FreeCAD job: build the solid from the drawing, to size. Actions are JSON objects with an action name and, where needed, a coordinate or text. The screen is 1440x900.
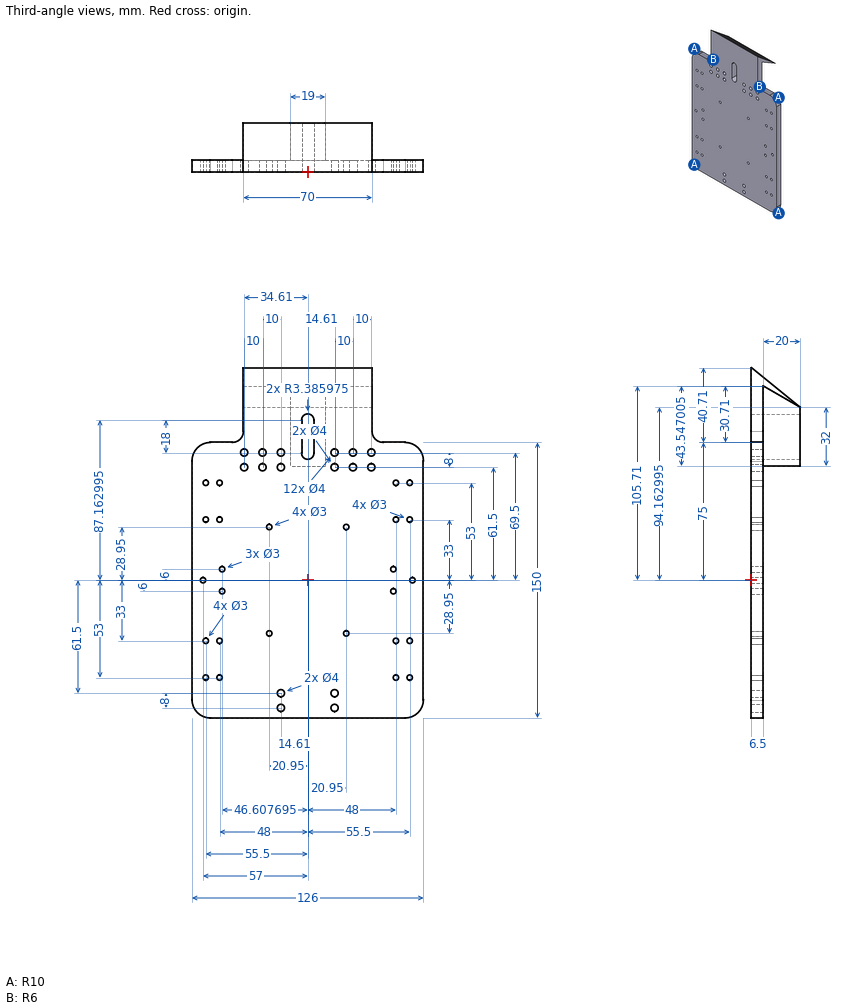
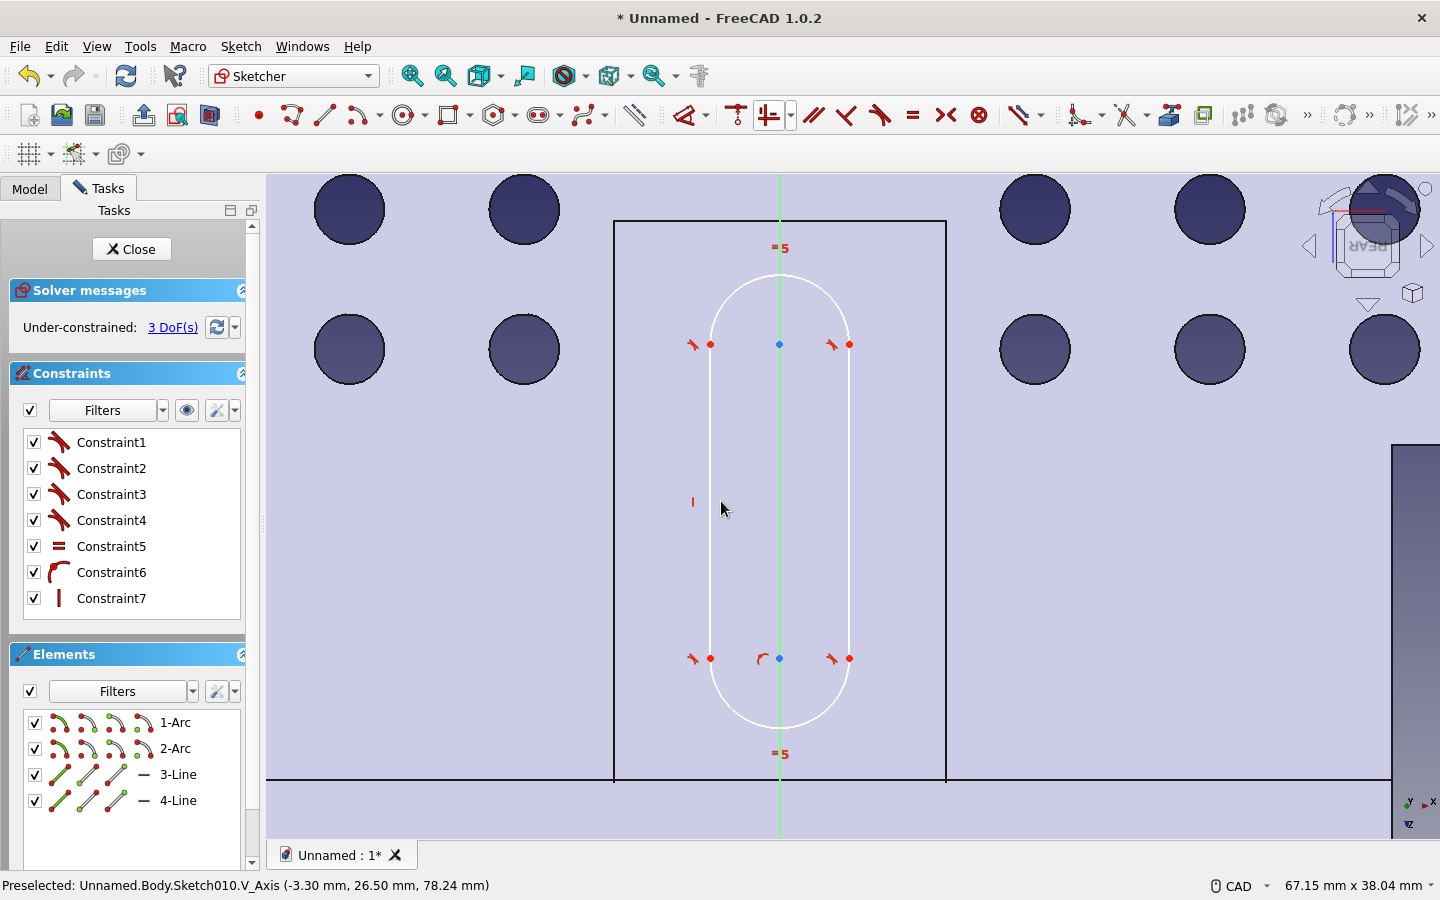
{"action": "left_click", "coordinate": [684, 116]}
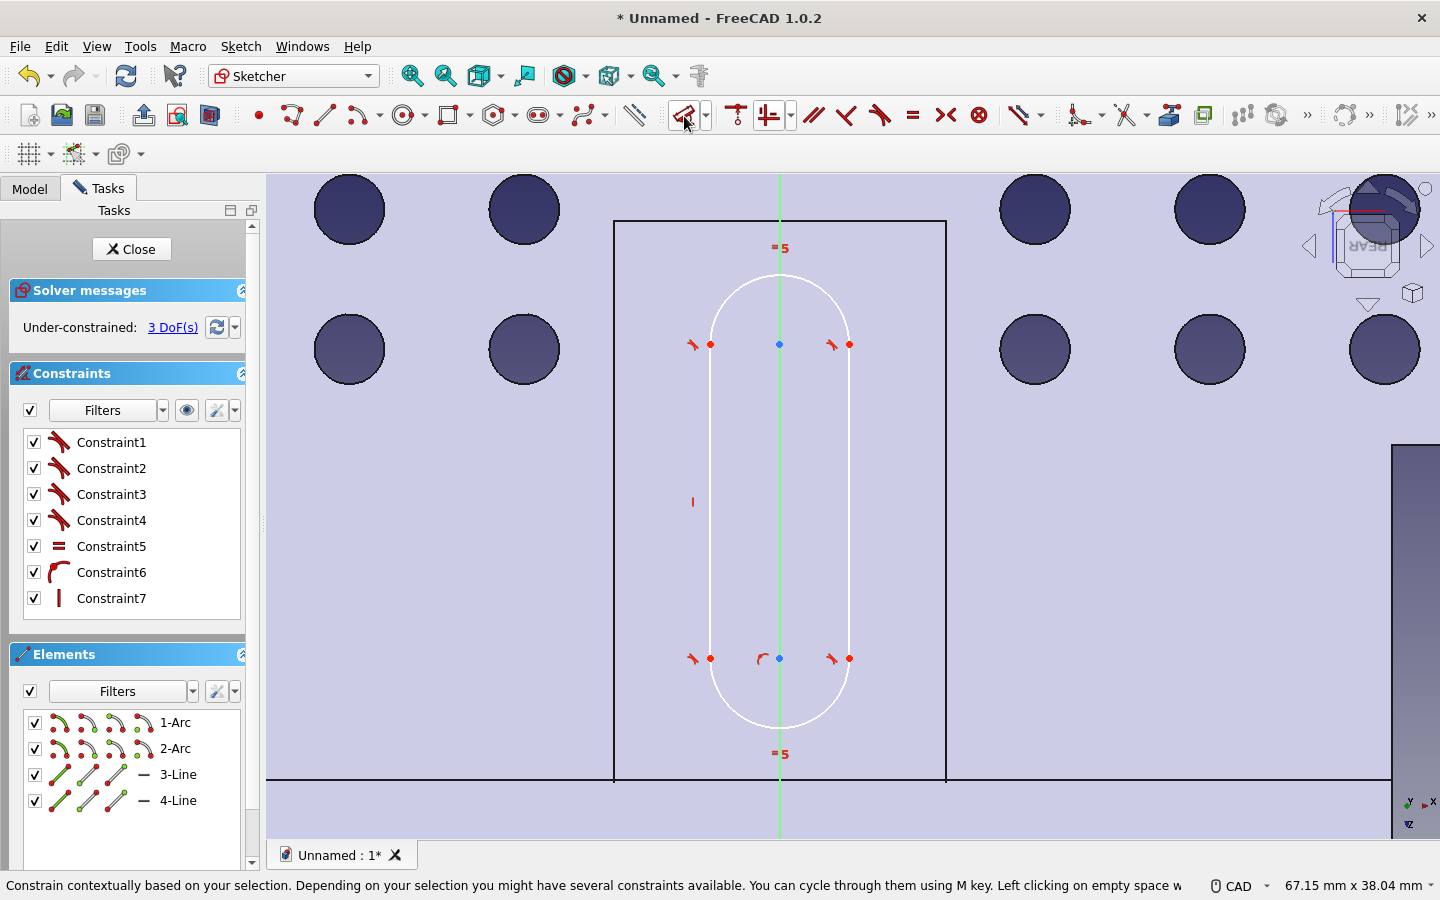
{"action": "left_click", "coordinate": [739, 715]}
{"action": "left_click", "coordinate": [720, 741]}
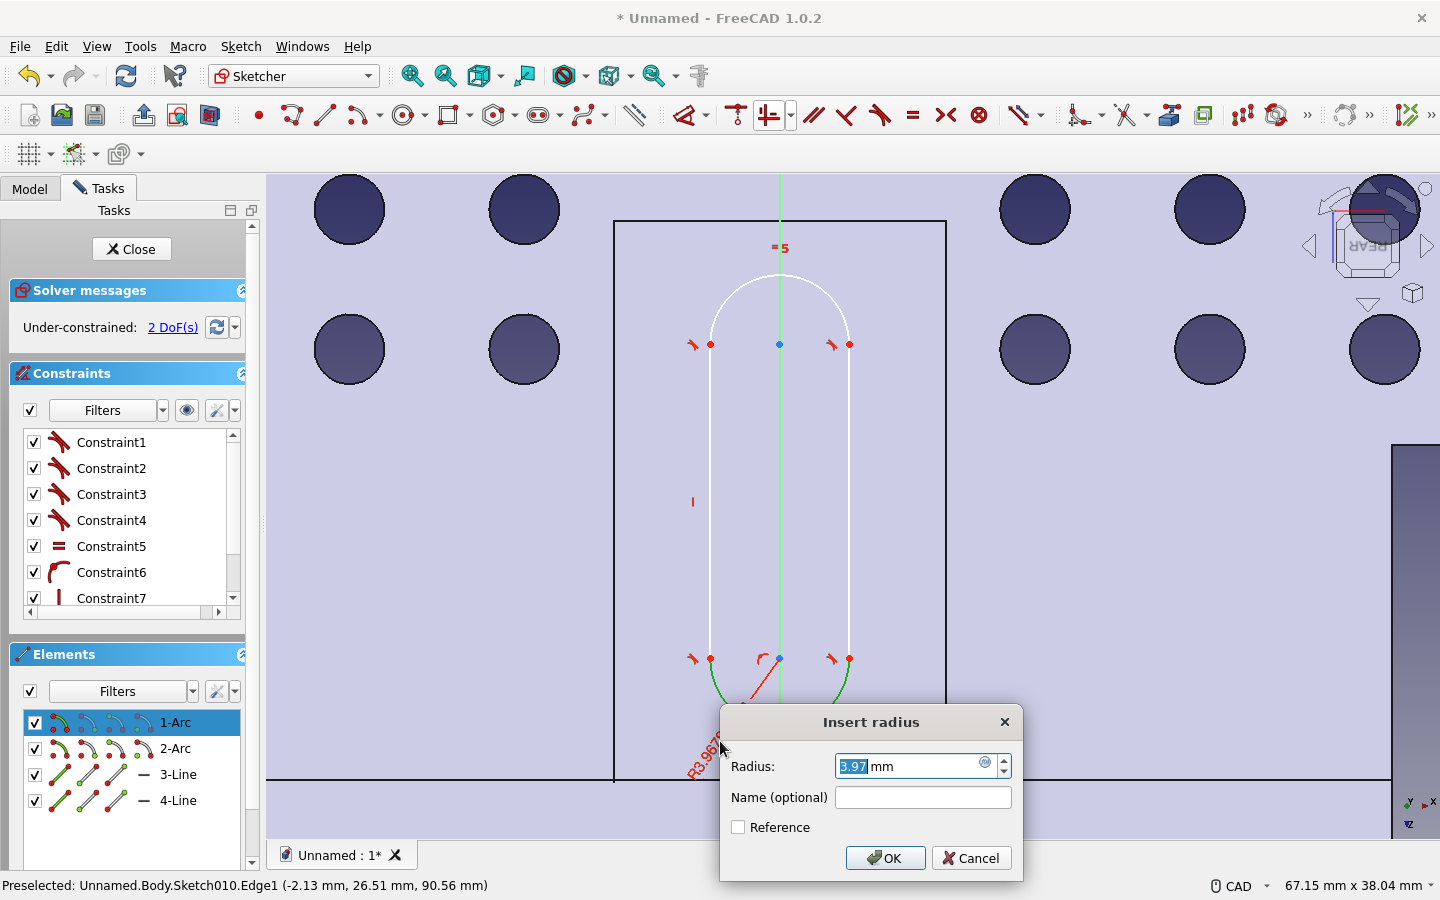
{"action": "type", "text": "3.385975"}
{"action": "key", "text": "Return"}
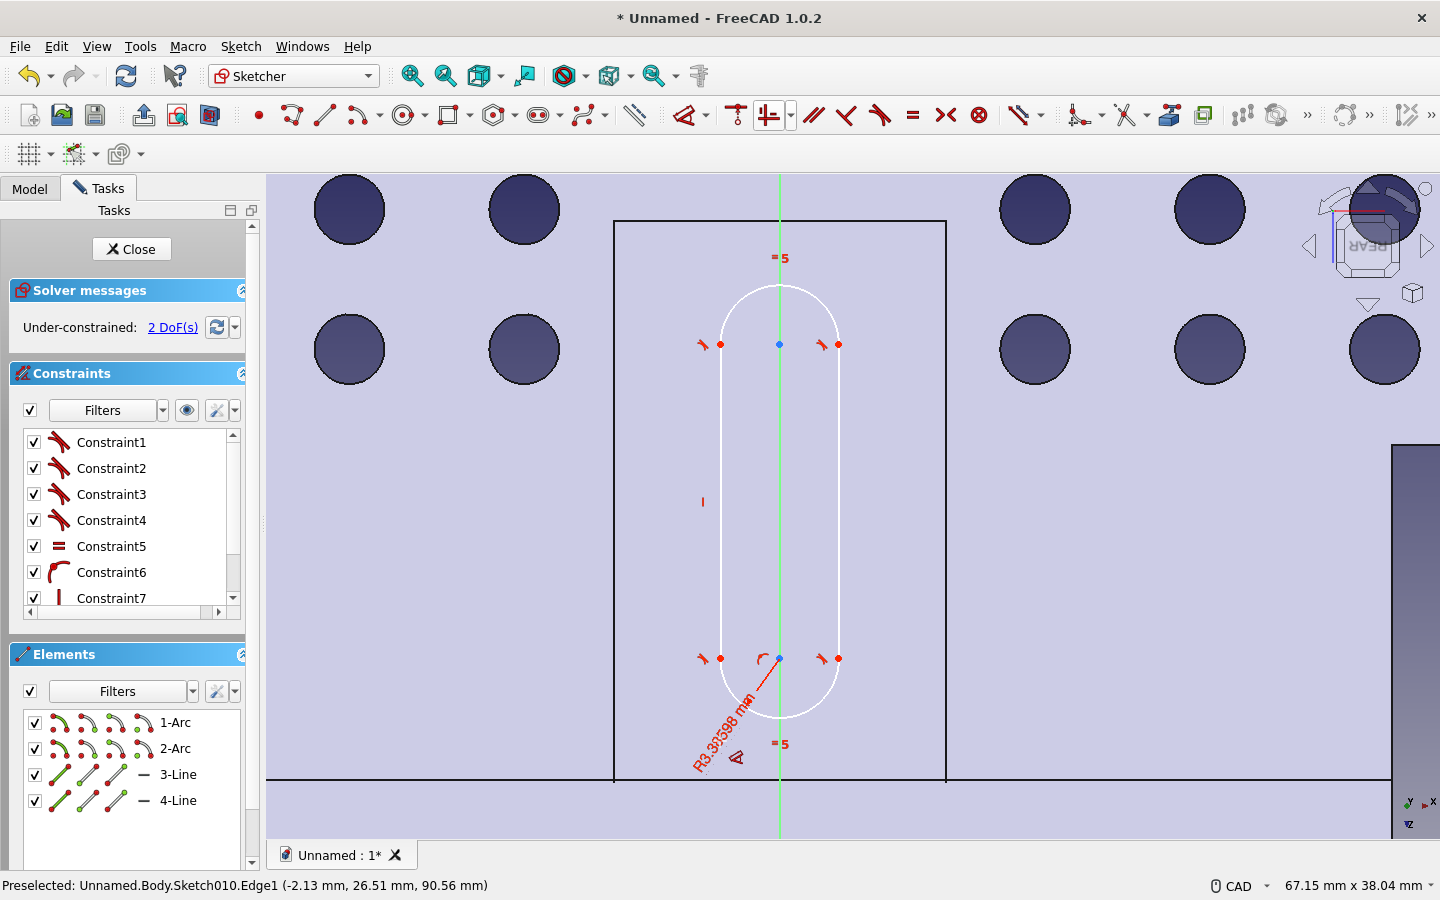
{"action": "left_click", "coordinate": [721, 565]}
{"action": "left_click", "coordinate": [687, 502]}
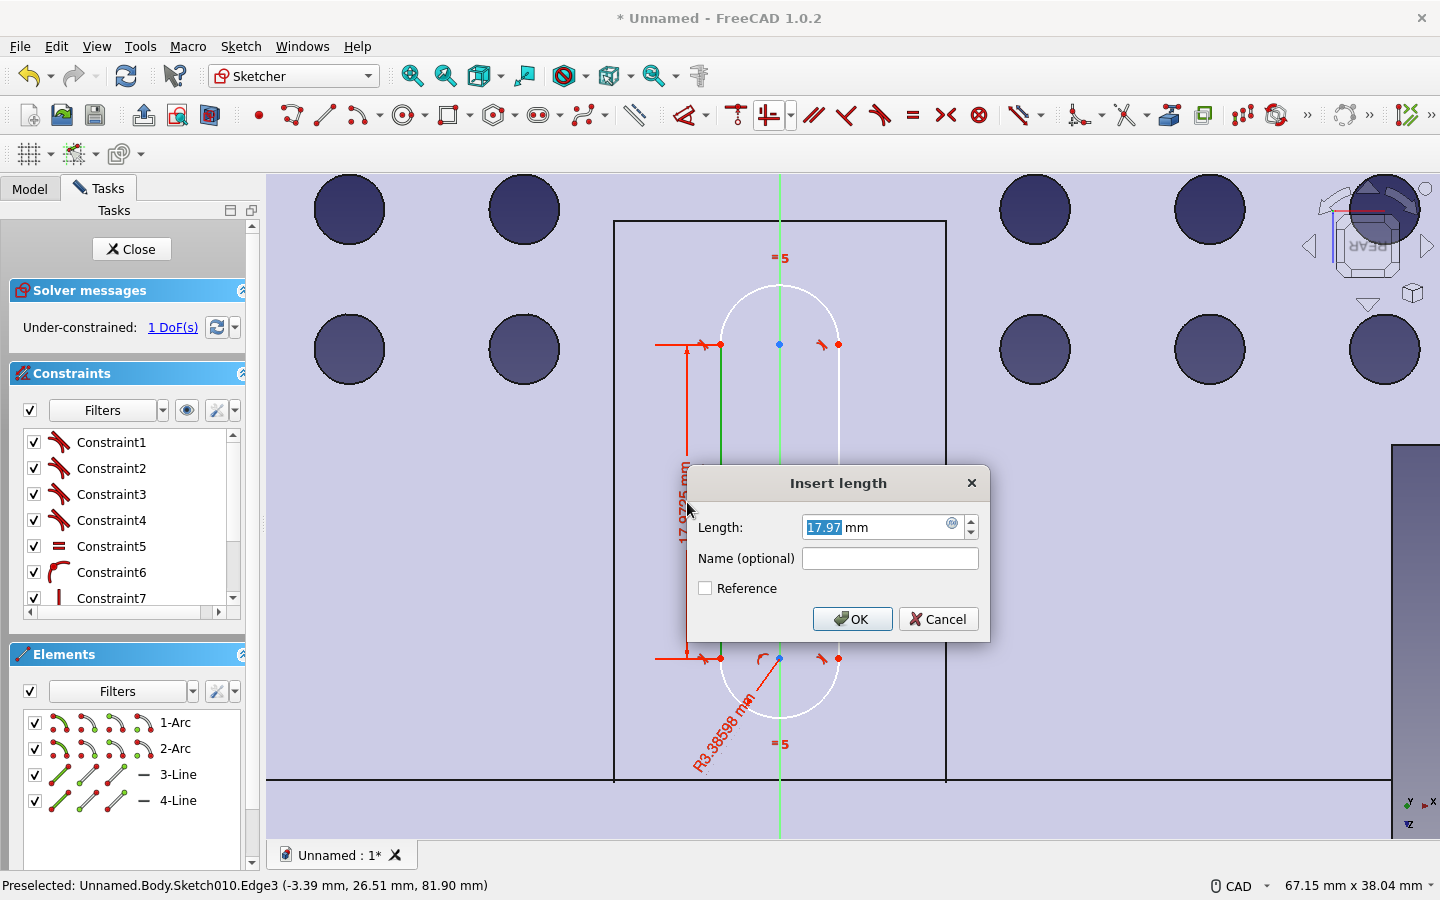
{"action": "type", "text": "18"}
{"action": "key", "text": "Return"}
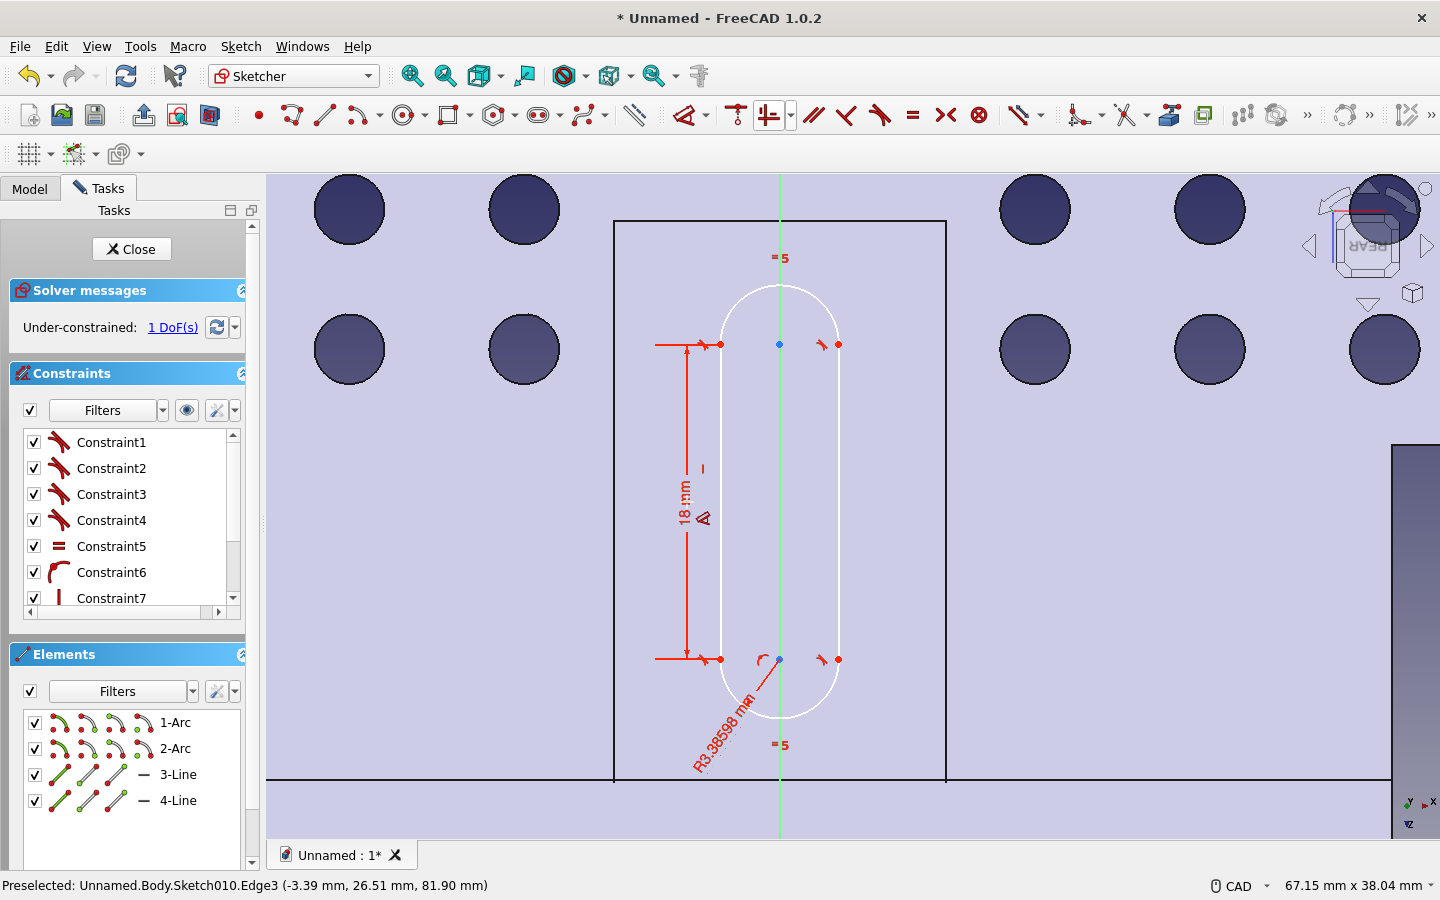
{"action": "left_click", "coordinate": [721, 659]}
{"action": "left_click", "coordinate": [687, 431]}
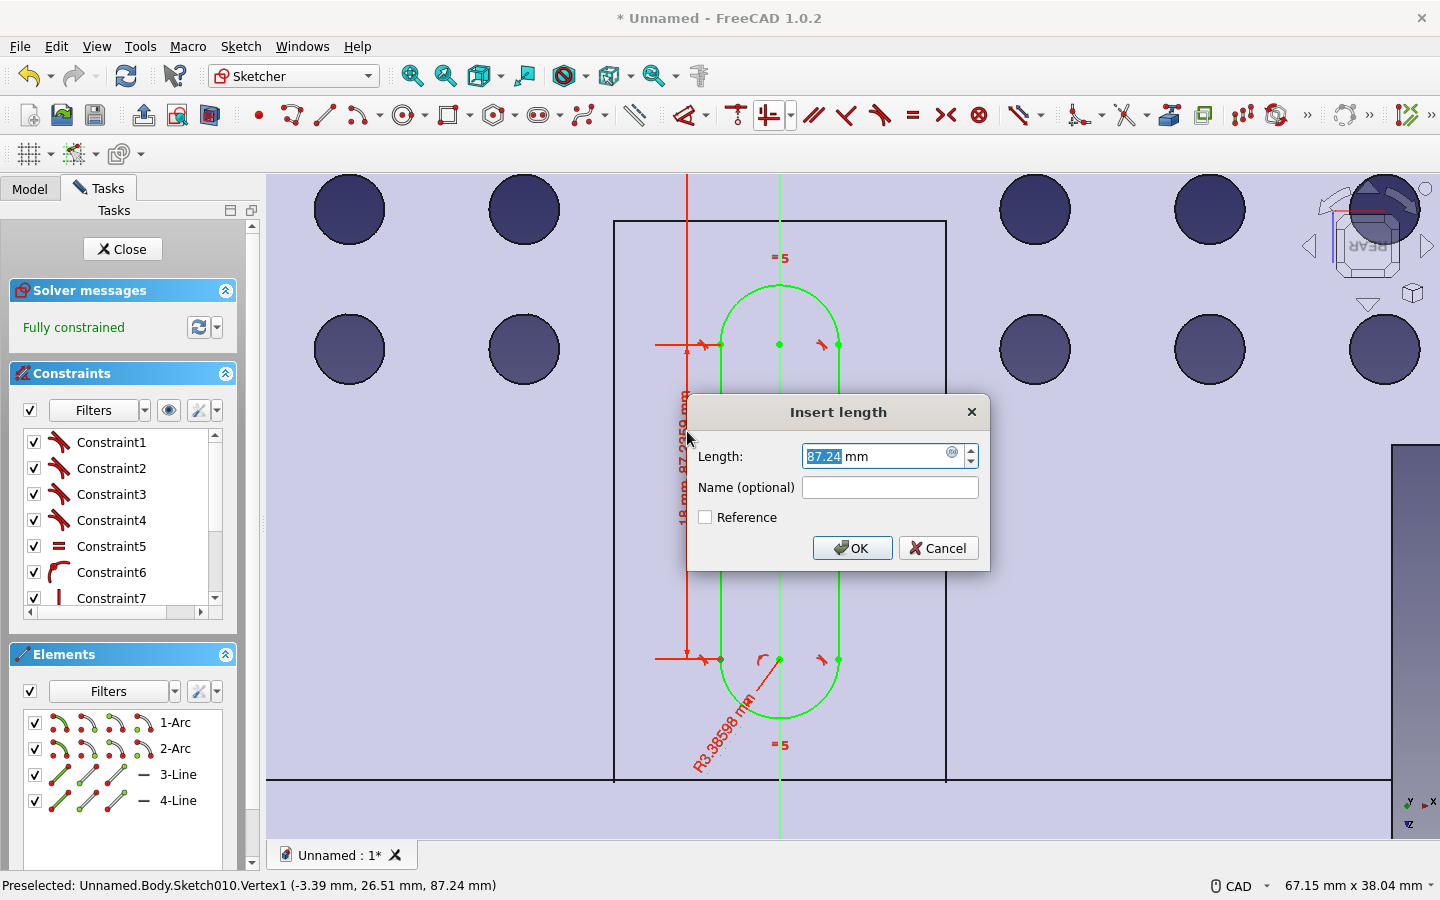
{"action": "type", "text": "87.162995"}
{"action": "key", "text": "Return"}
{"action": "key", "text": "Escape"}